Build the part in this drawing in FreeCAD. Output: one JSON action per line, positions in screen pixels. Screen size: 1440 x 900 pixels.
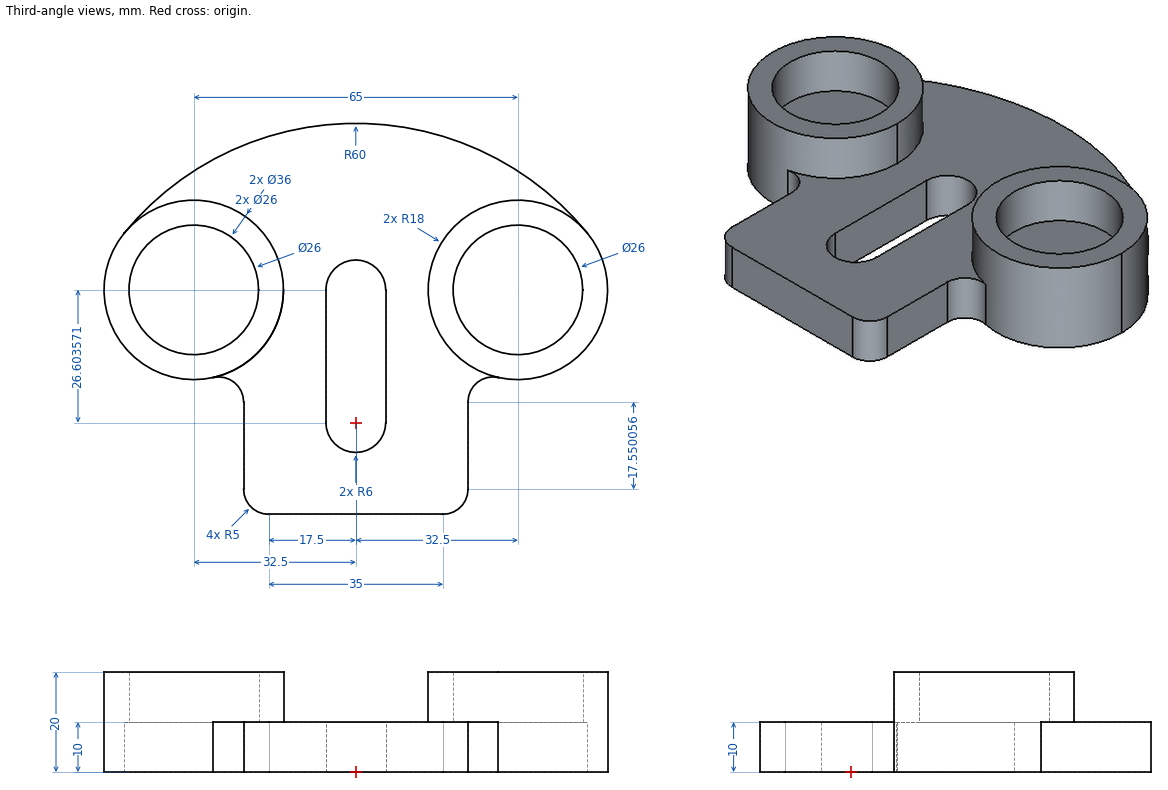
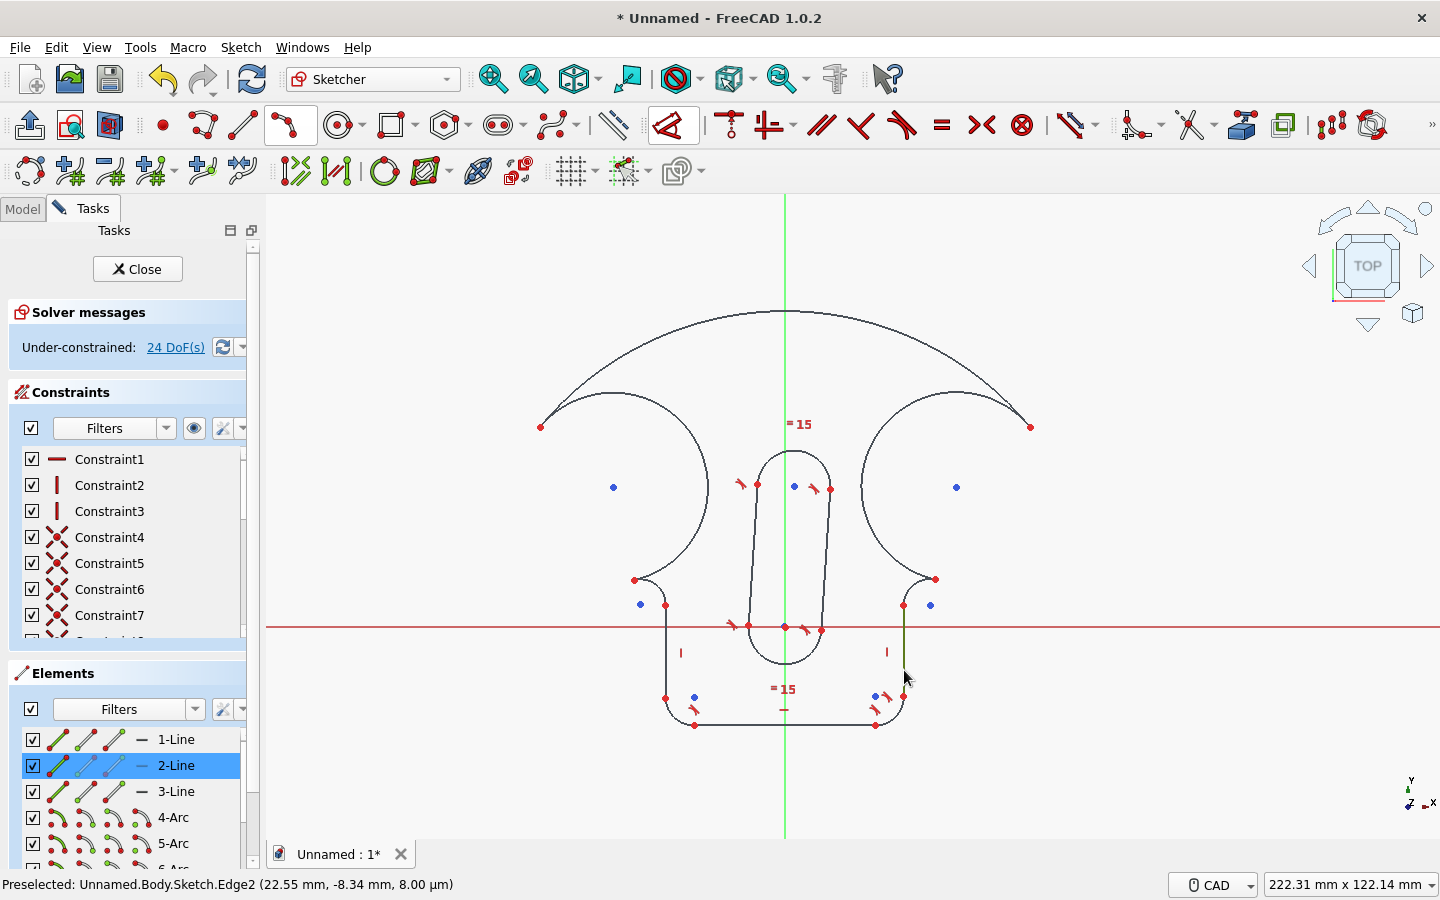
{"action": "left_click", "coordinate": [907, 592]}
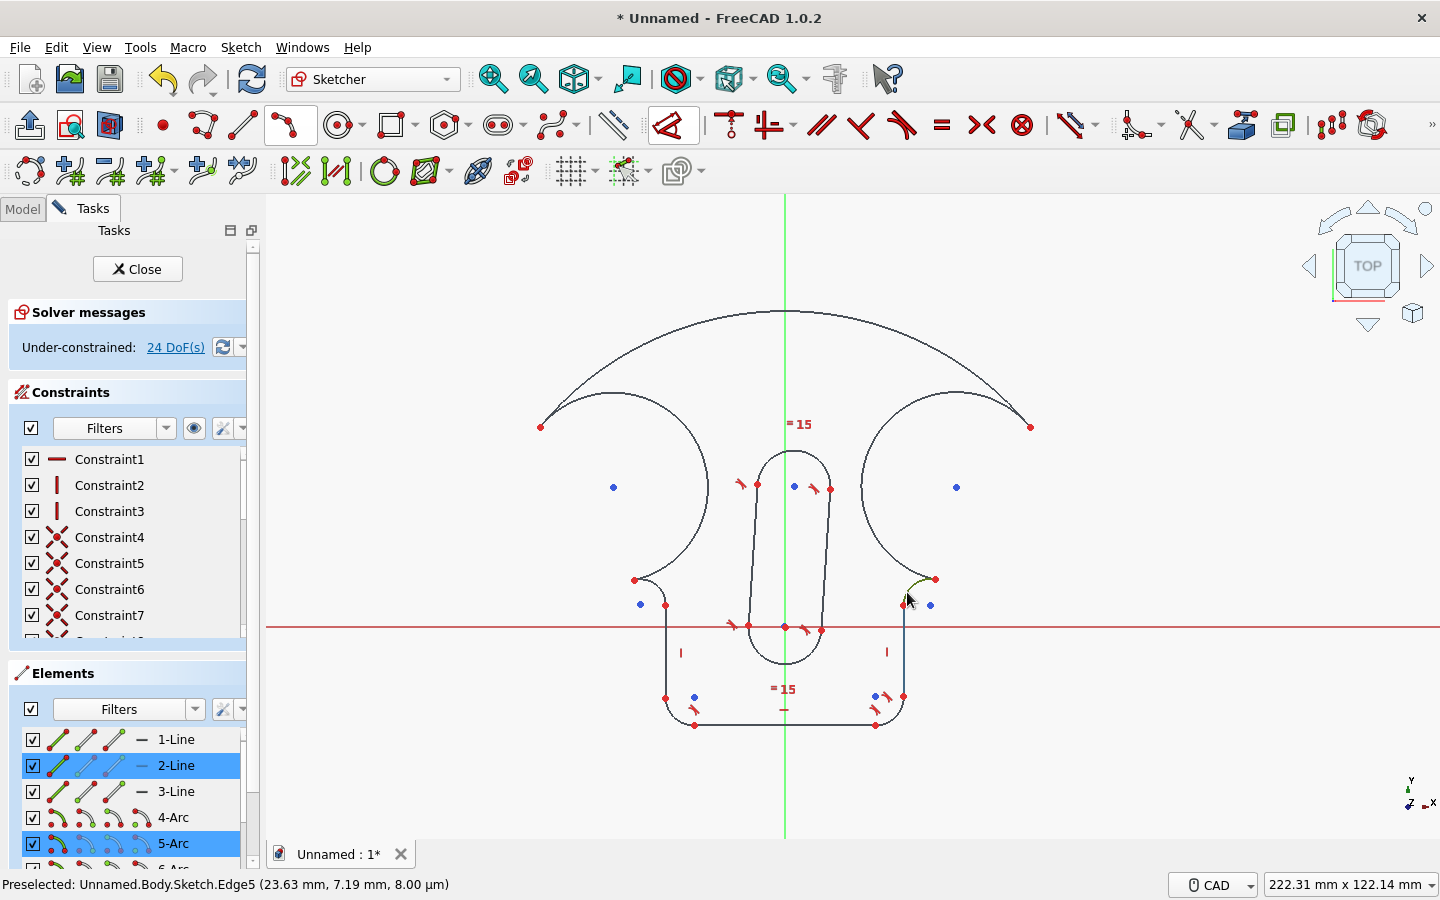
{"action": "left_click", "coordinate": [902, 126]}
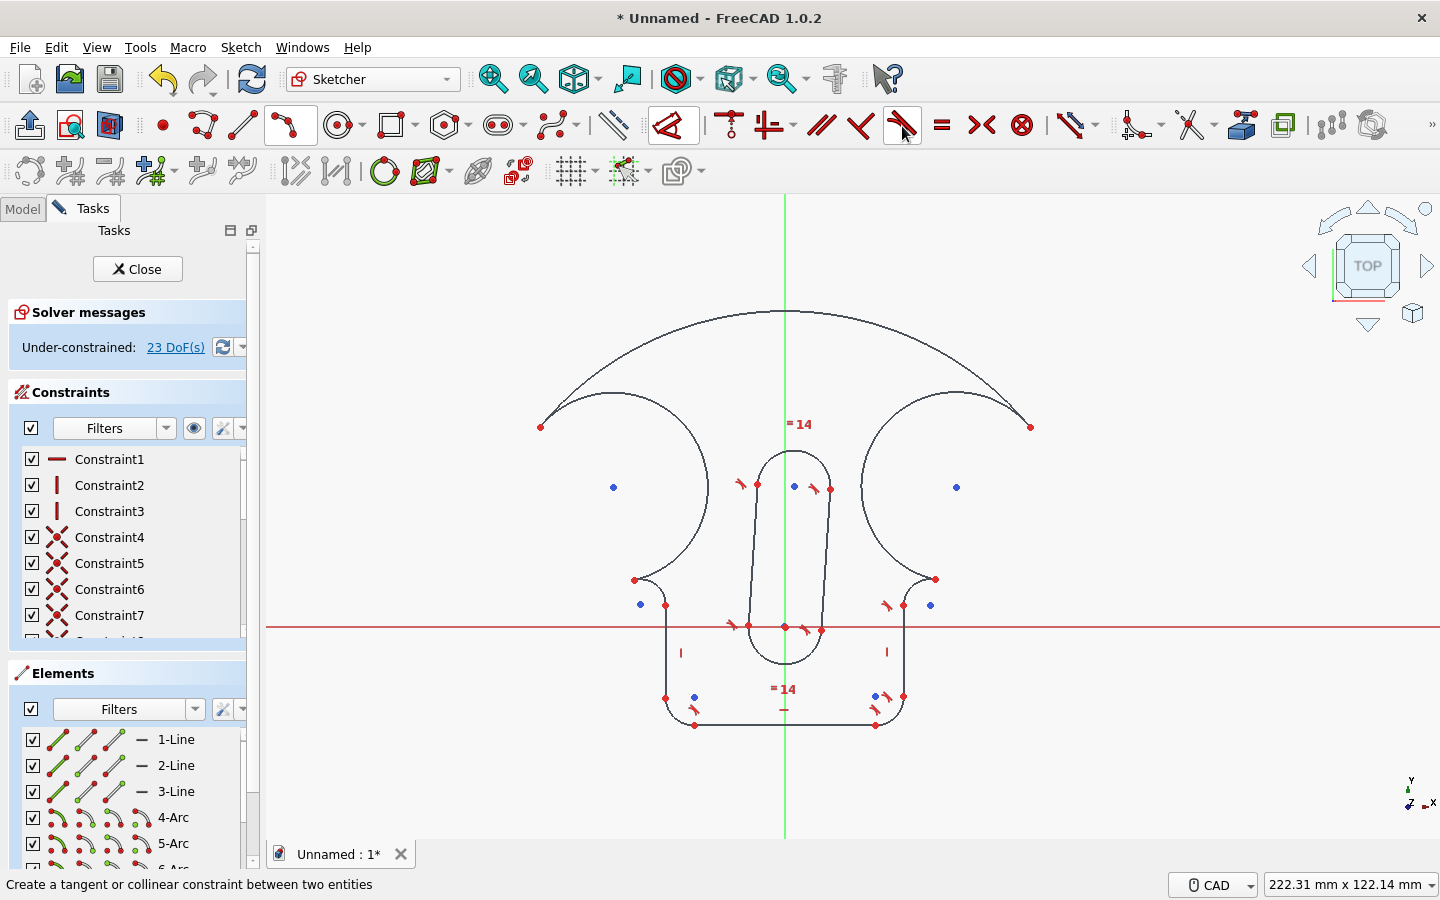
{"action": "left_click", "coordinate": [666, 671]}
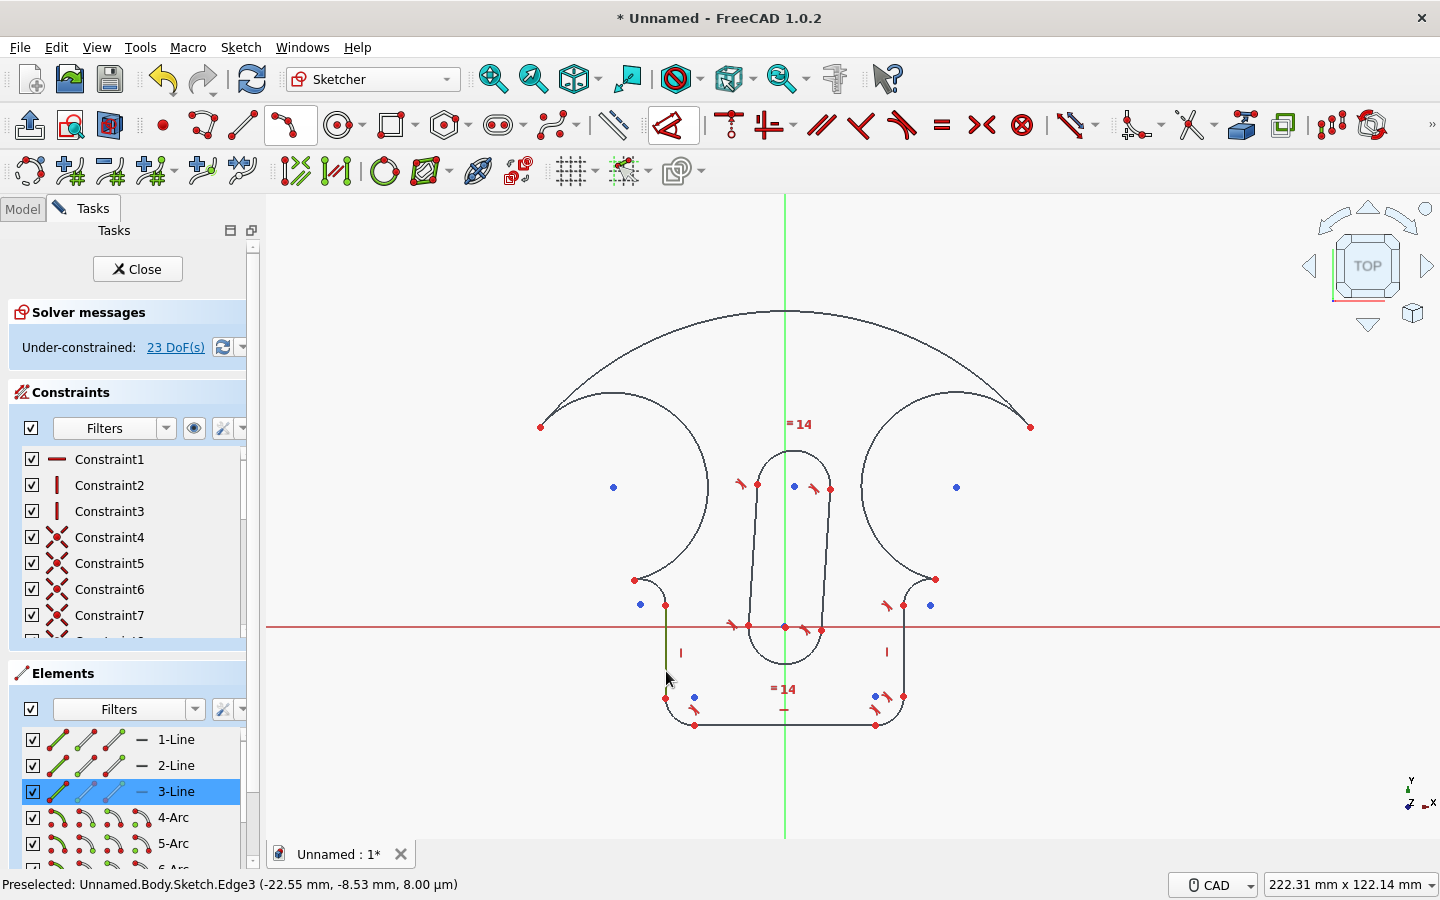
{"action": "left_click", "coordinate": [662, 592]}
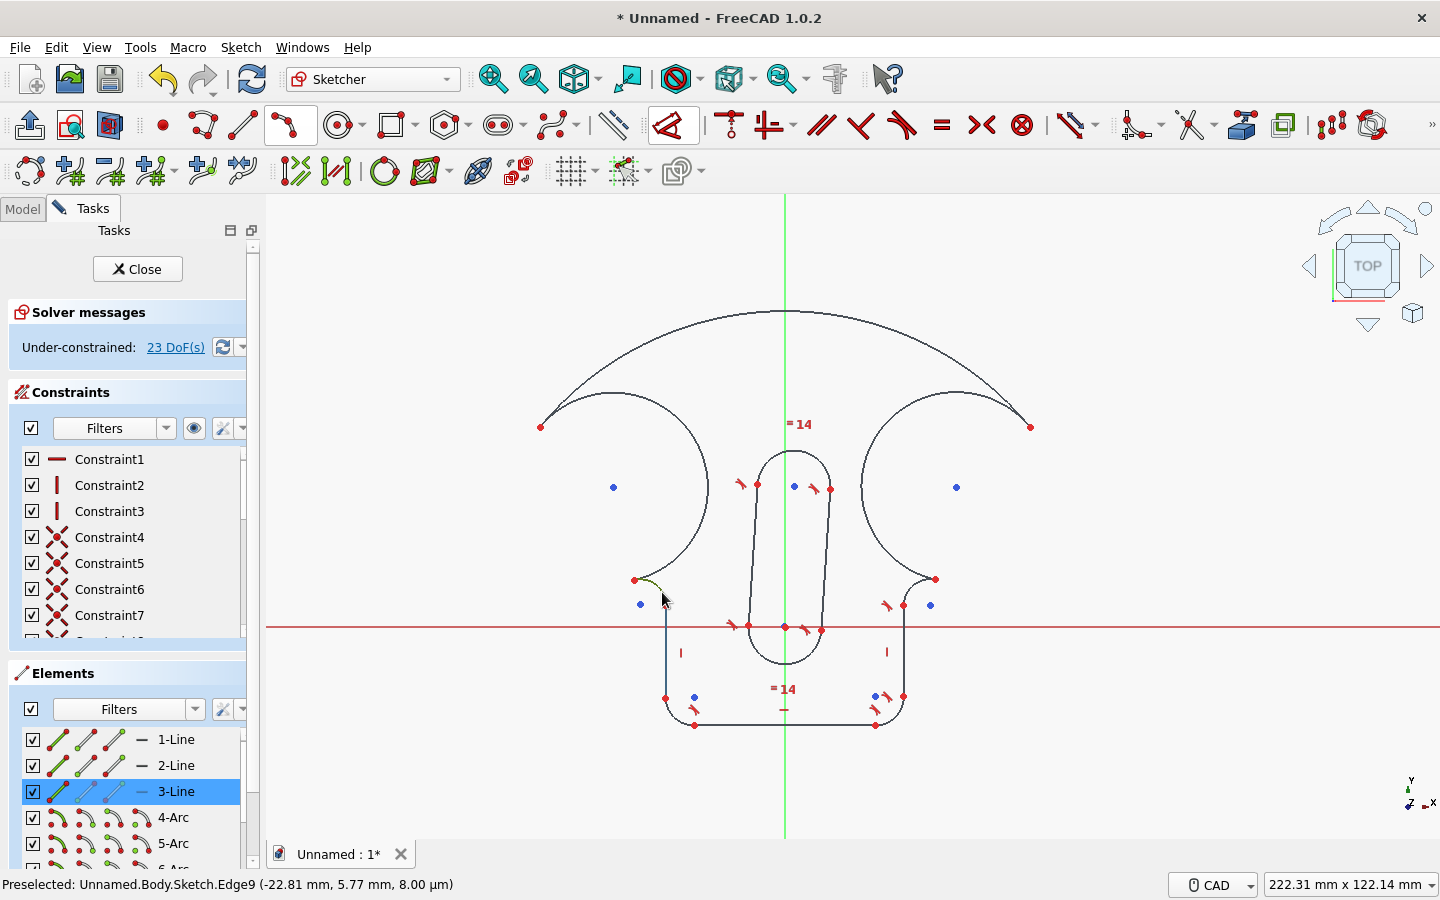
{"action": "left_click", "coordinate": [902, 126]}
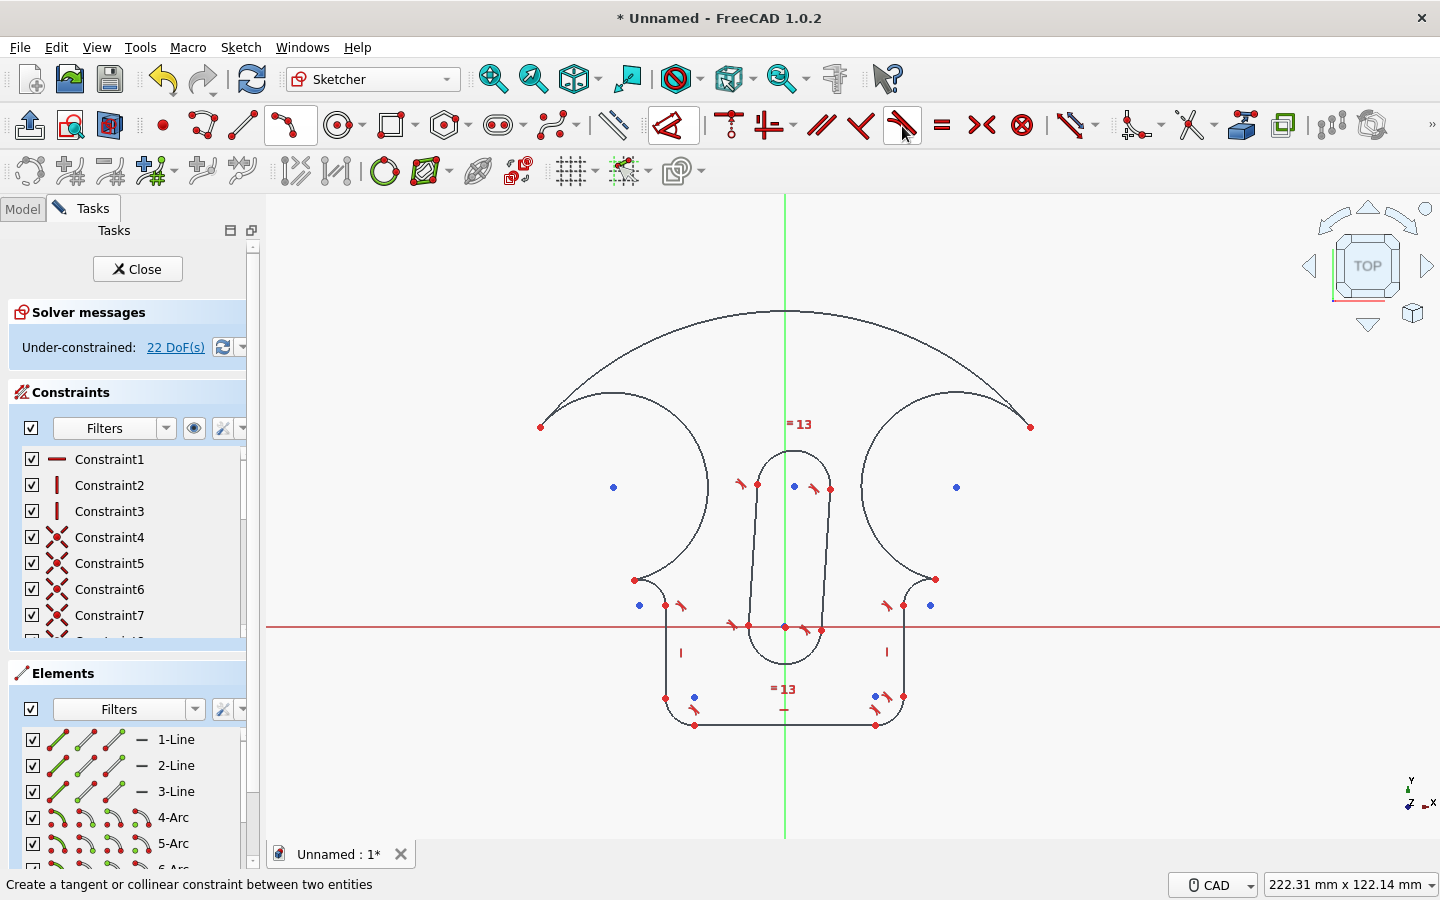
{"action": "left_click", "coordinate": [666, 671]}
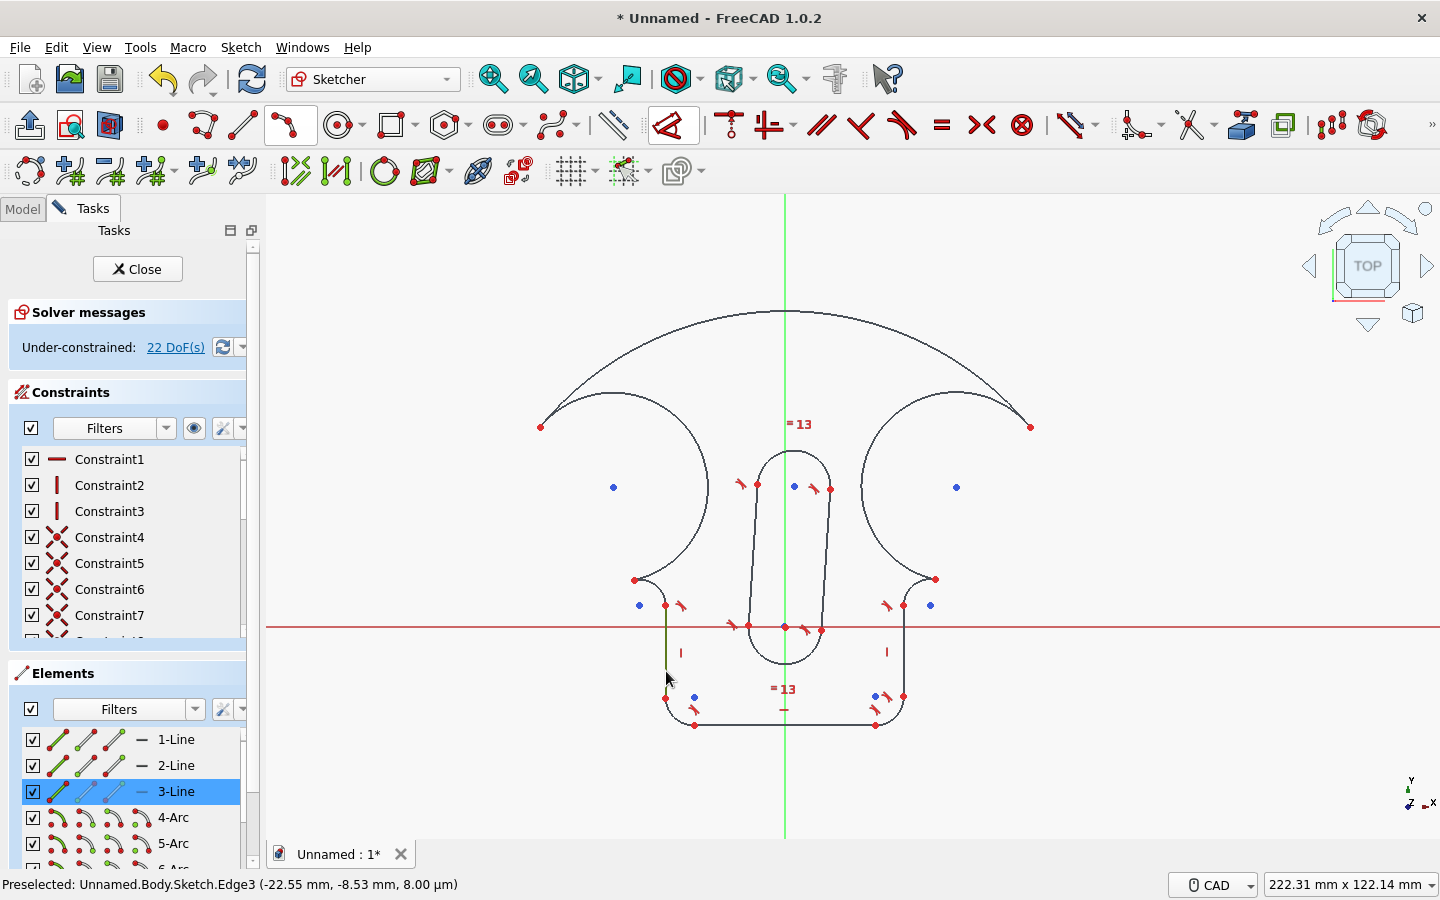
{"action": "left_click", "coordinate": [669, 711]}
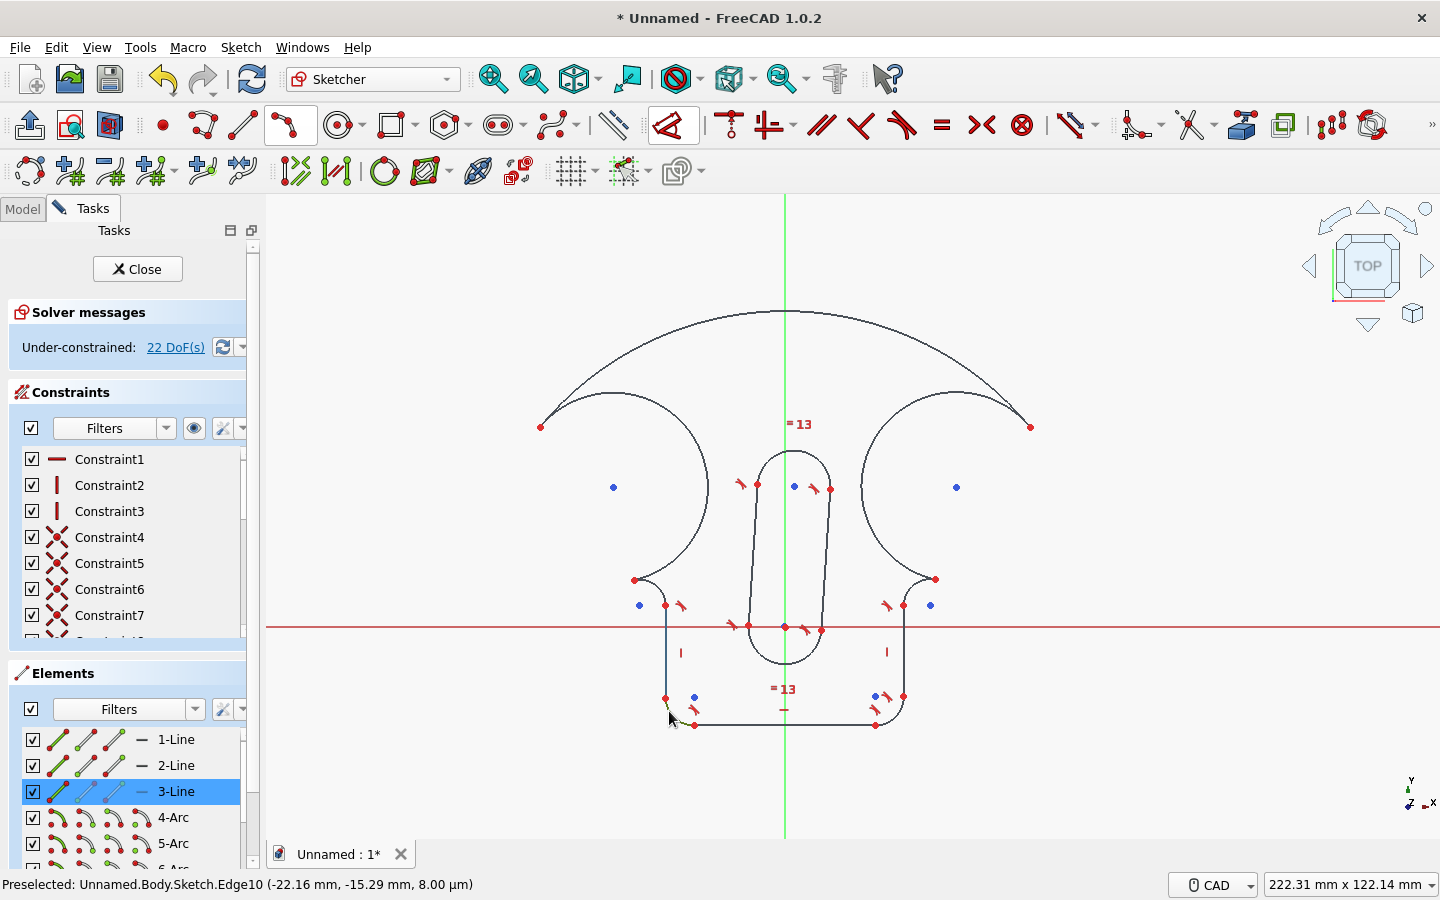
{"action": "left_click", "coordinate": [902, 126]}